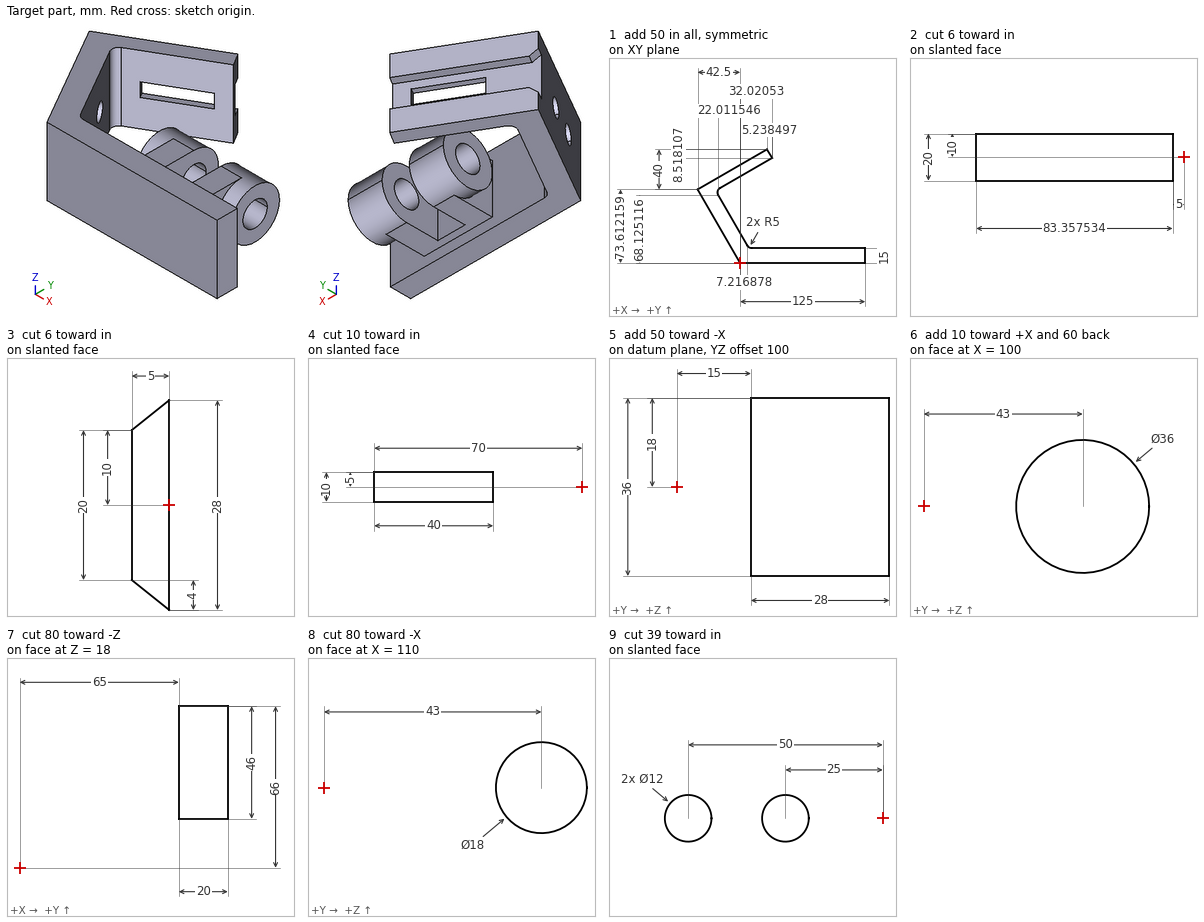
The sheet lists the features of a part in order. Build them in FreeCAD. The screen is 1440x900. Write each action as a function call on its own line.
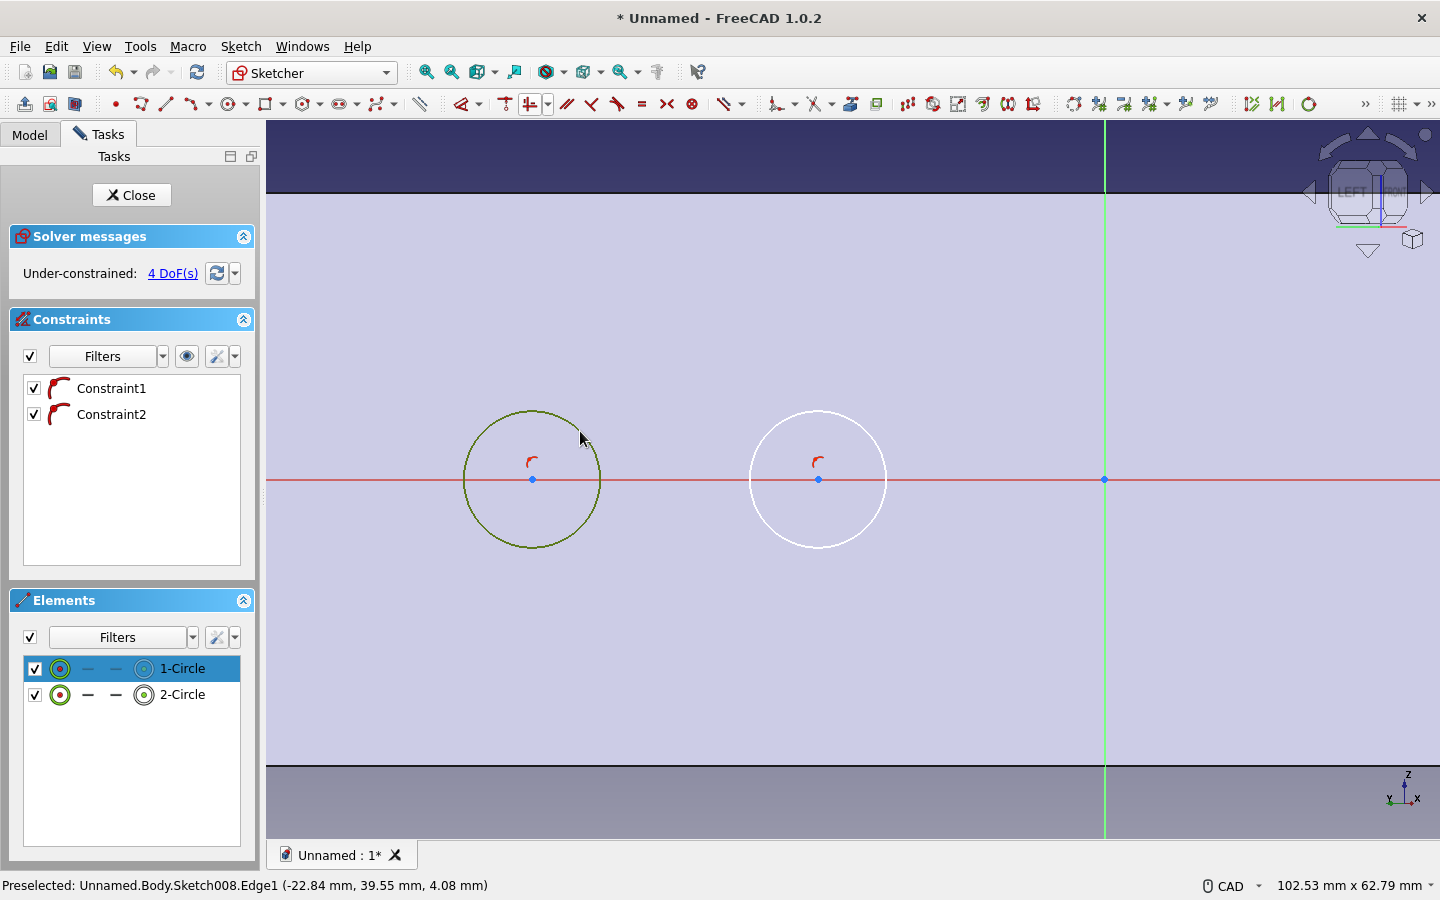
click(866, 431)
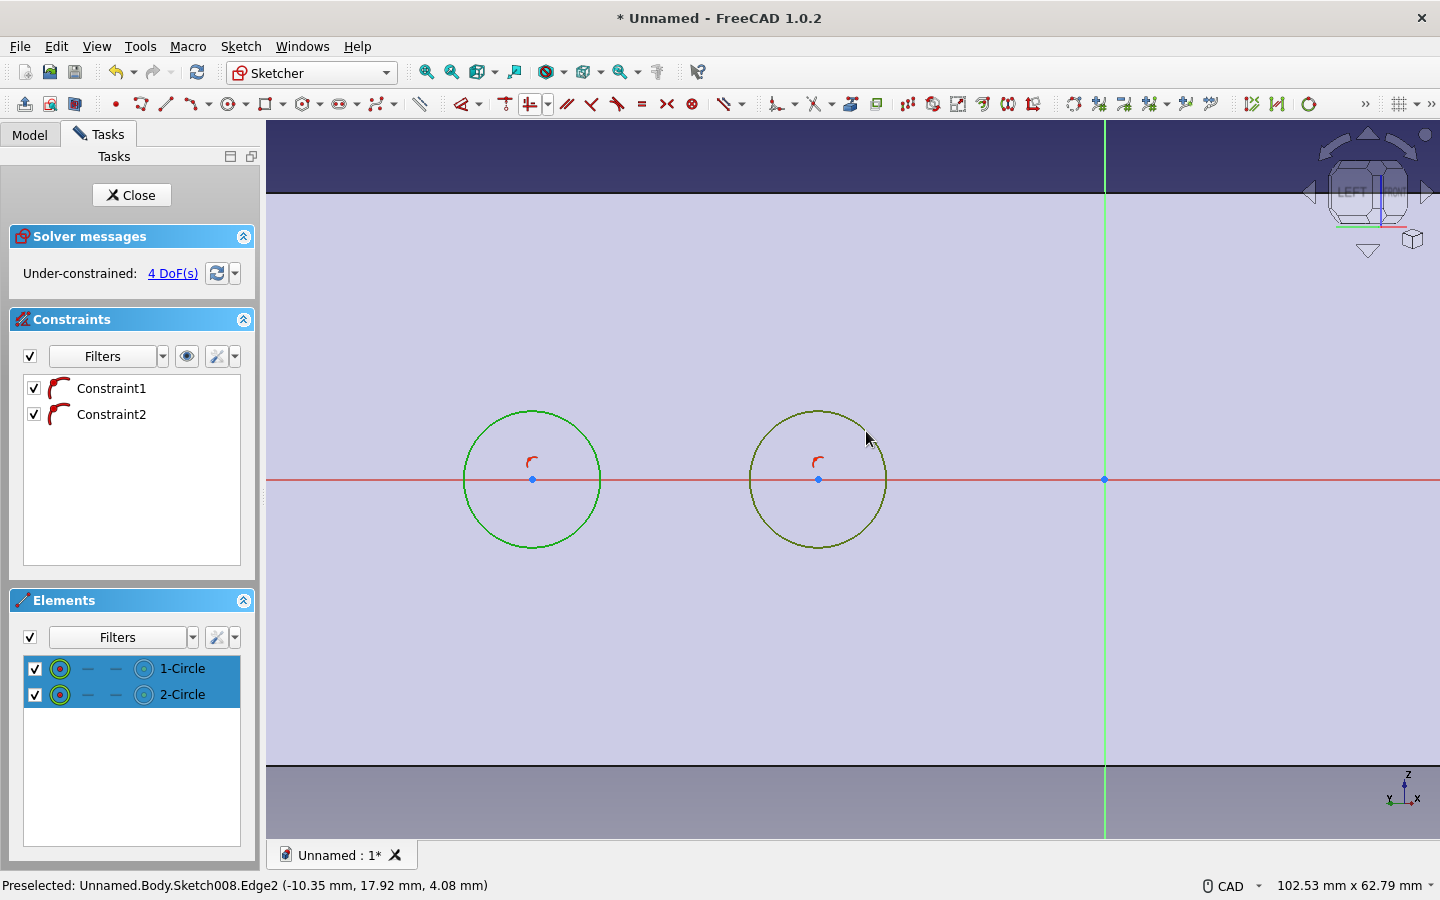
click(642, 104)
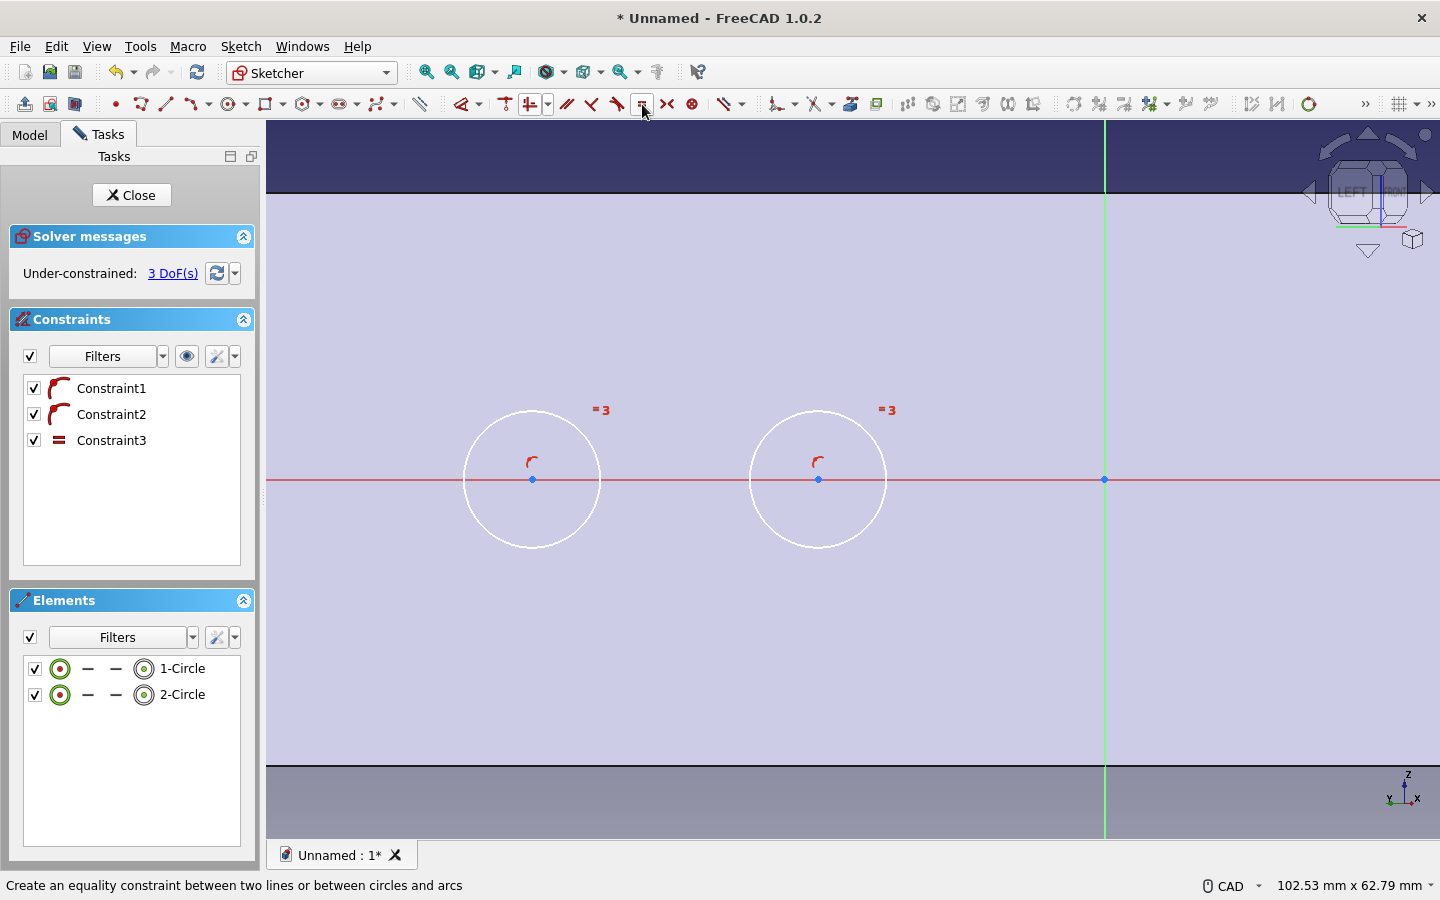
key(d)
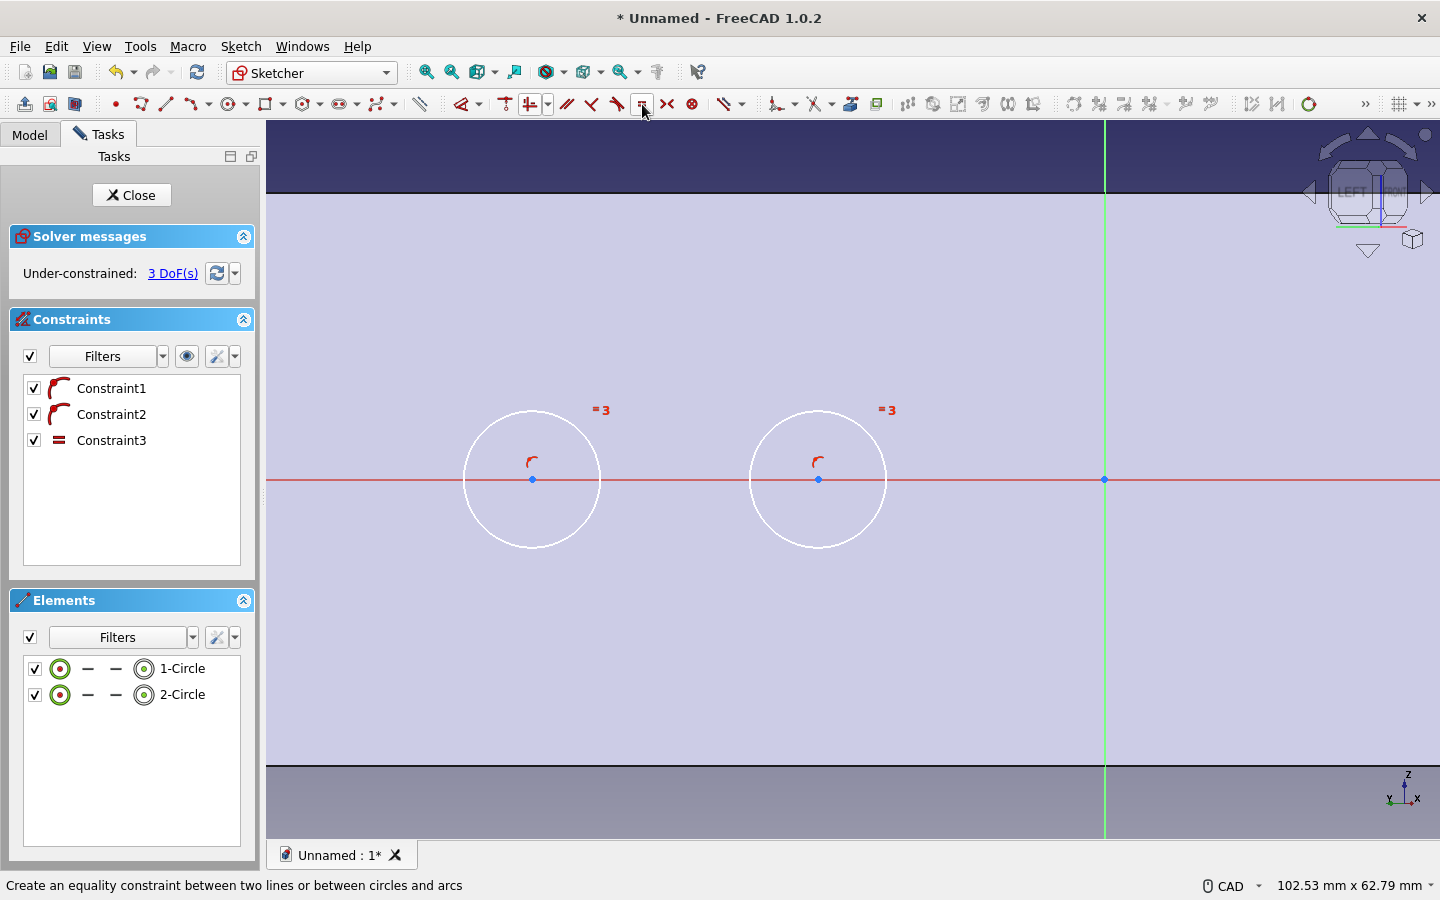
click(580, 431)
click(603, 408)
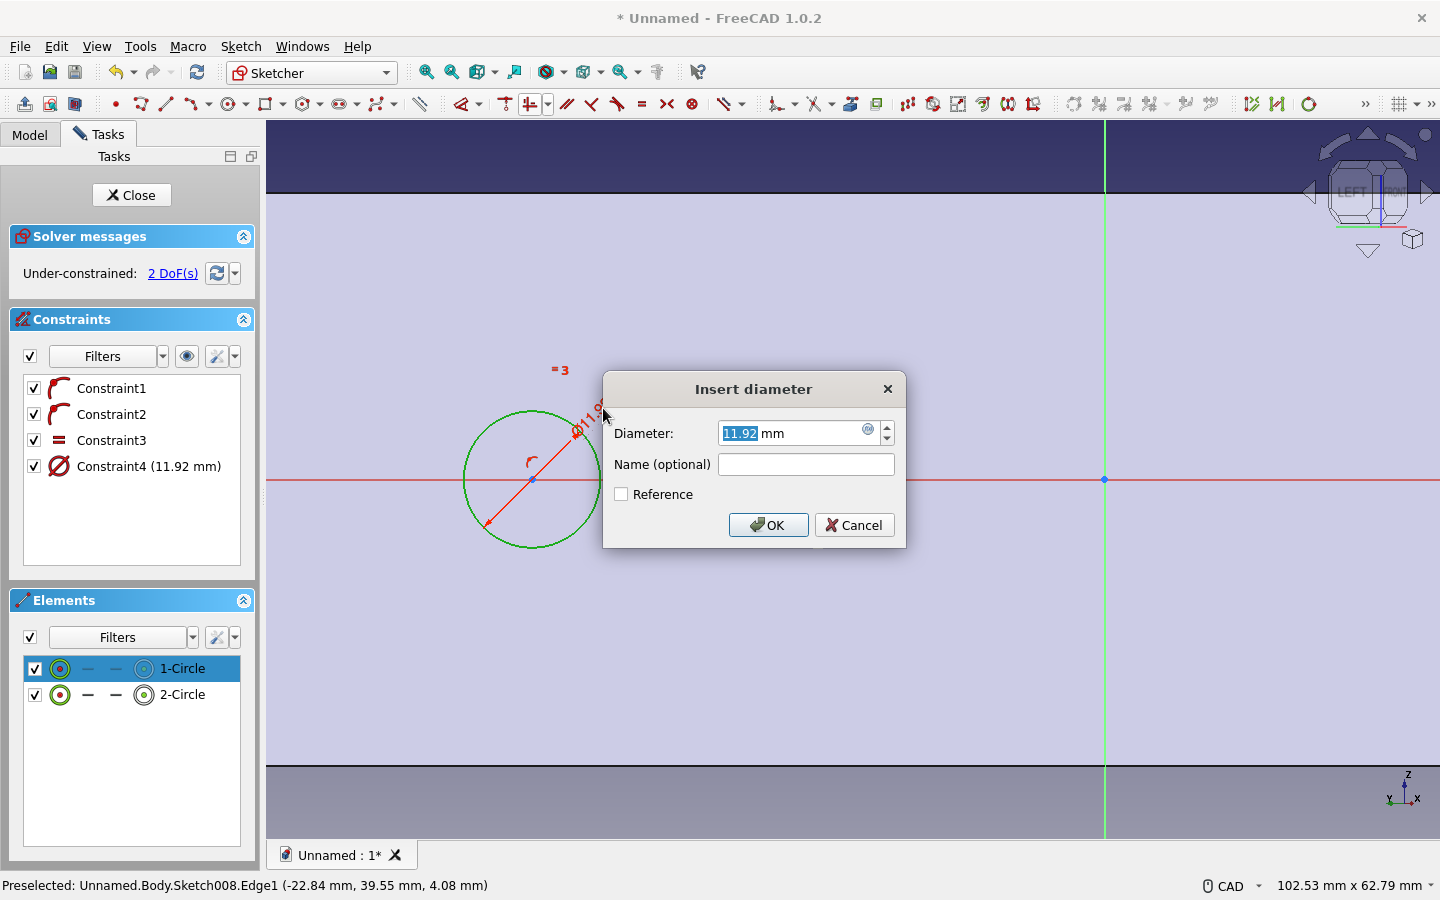
text(12)
key(Return)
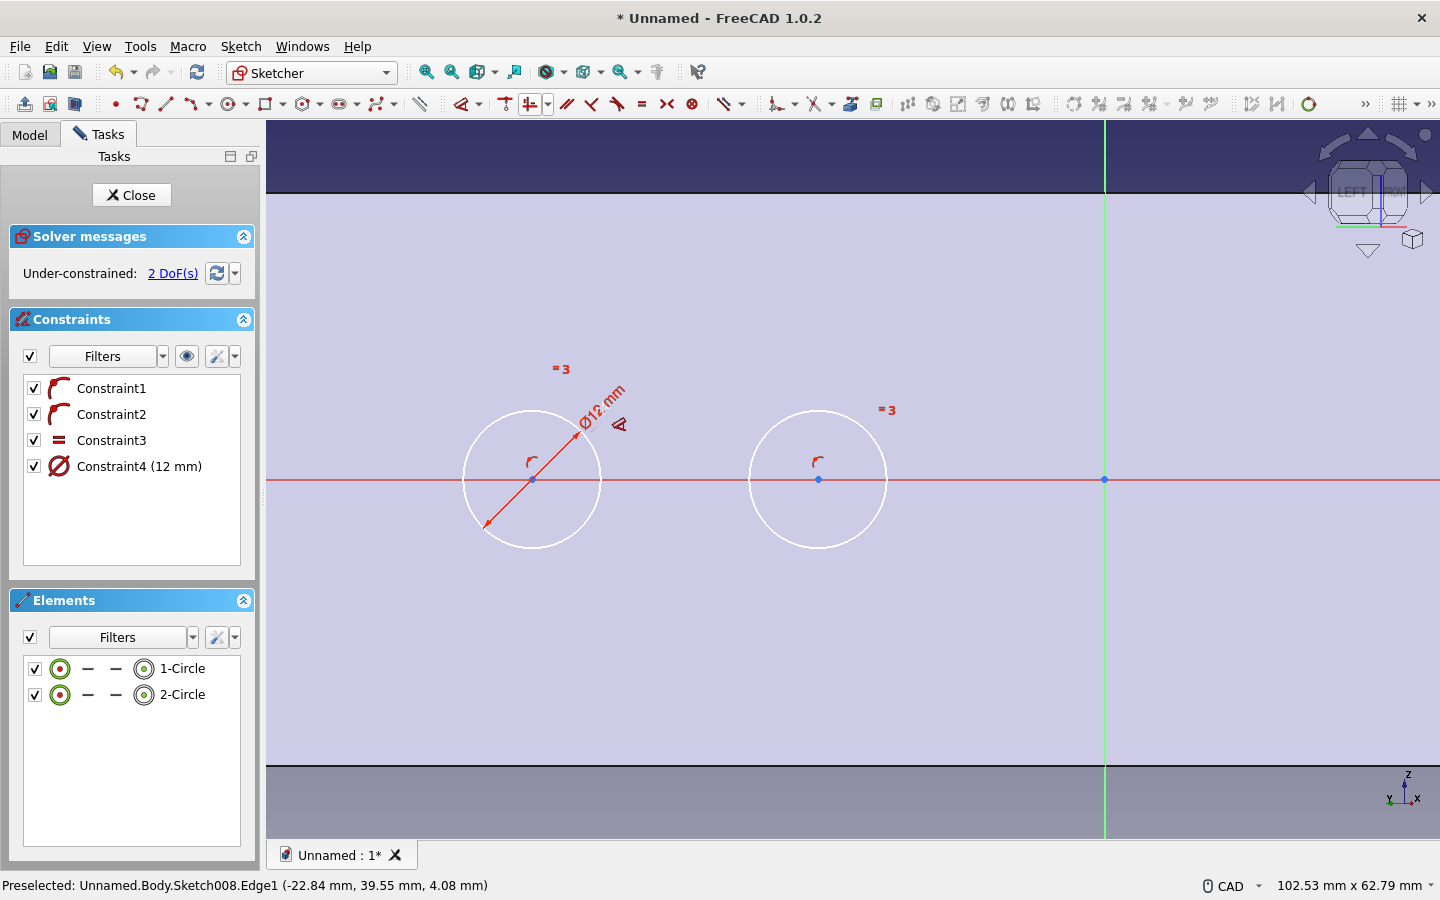
click(532, 479)
click(818, 513)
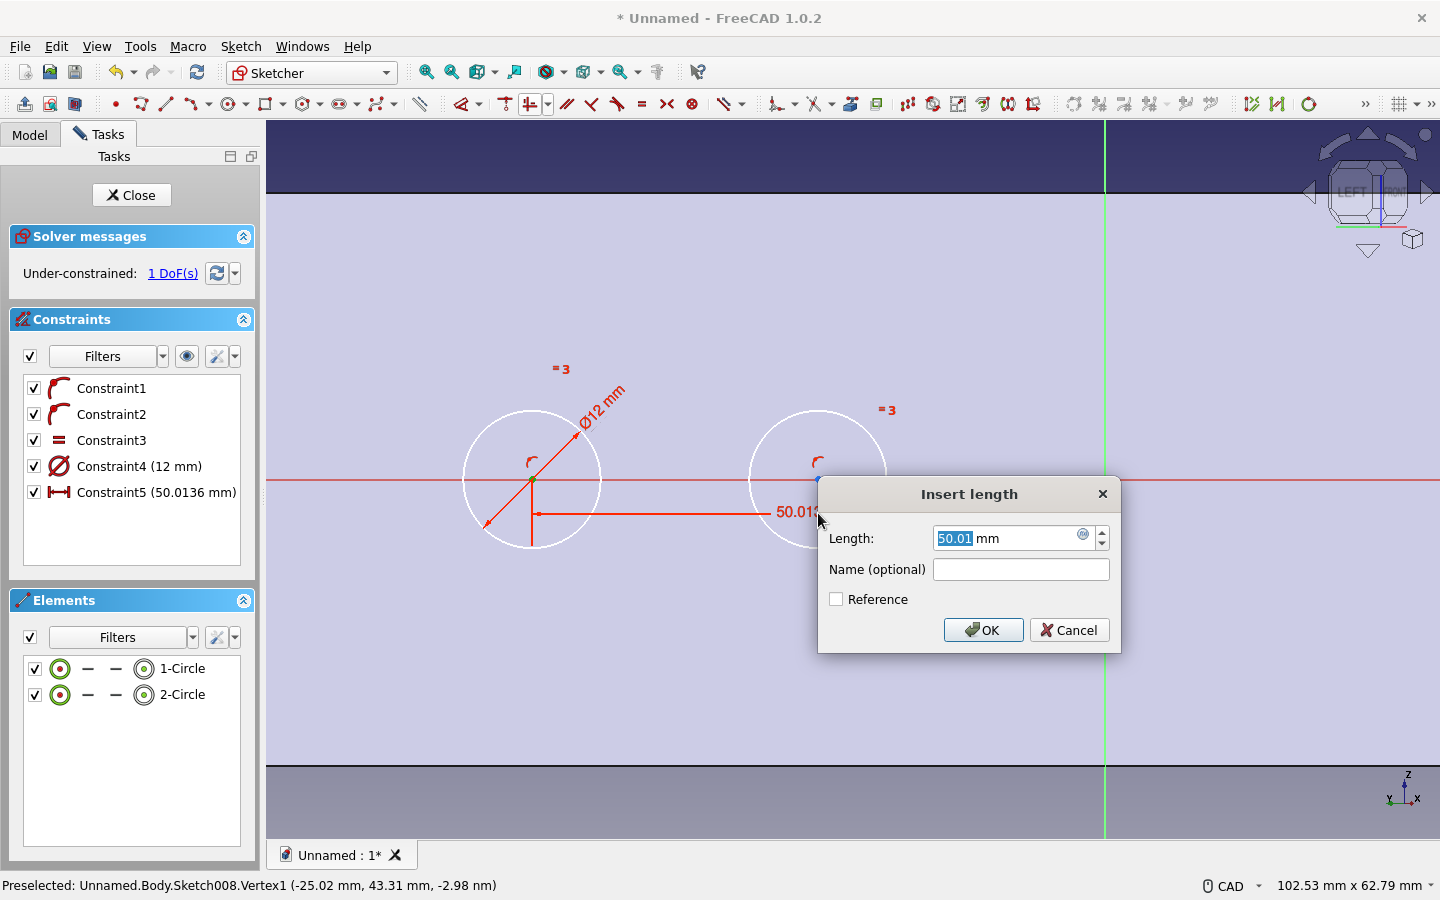
text(50)
key(Return)